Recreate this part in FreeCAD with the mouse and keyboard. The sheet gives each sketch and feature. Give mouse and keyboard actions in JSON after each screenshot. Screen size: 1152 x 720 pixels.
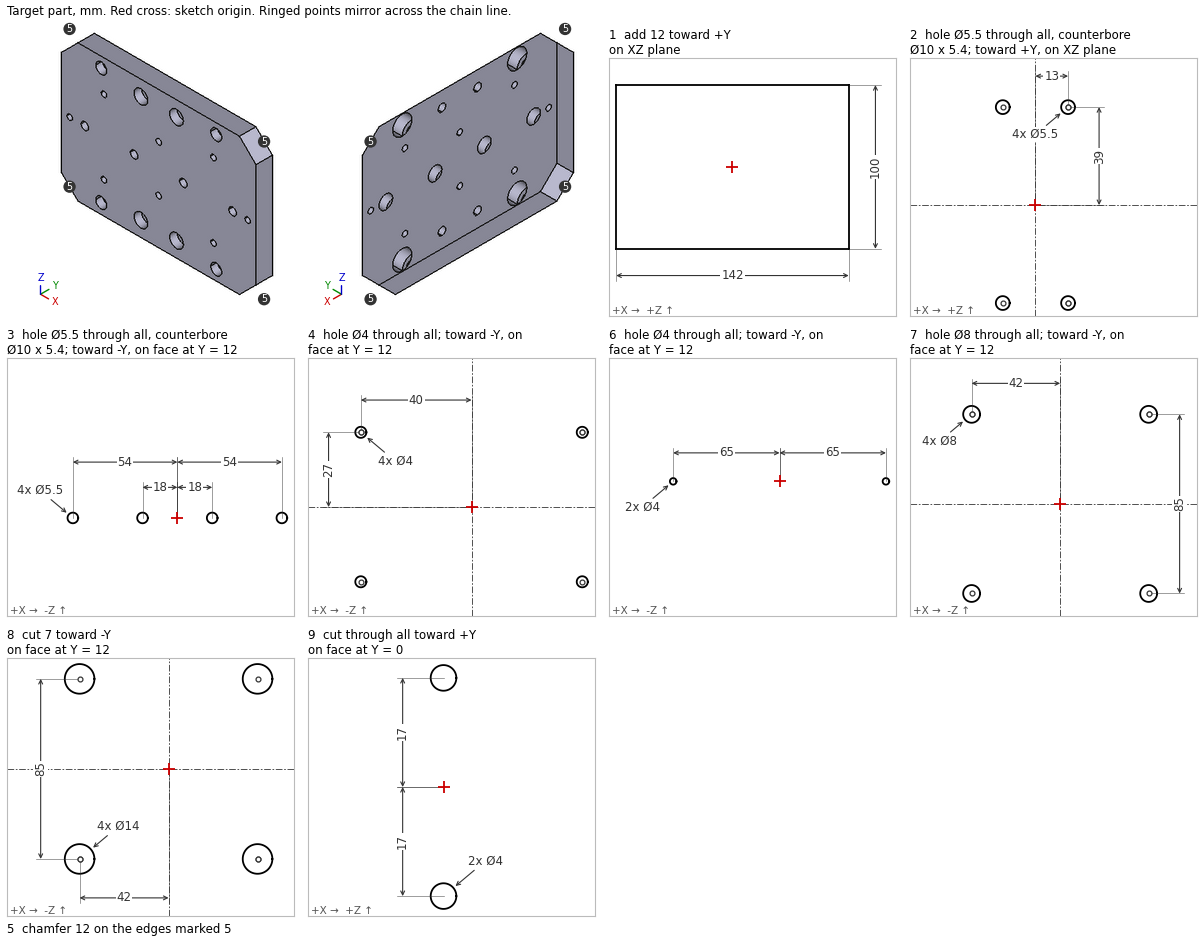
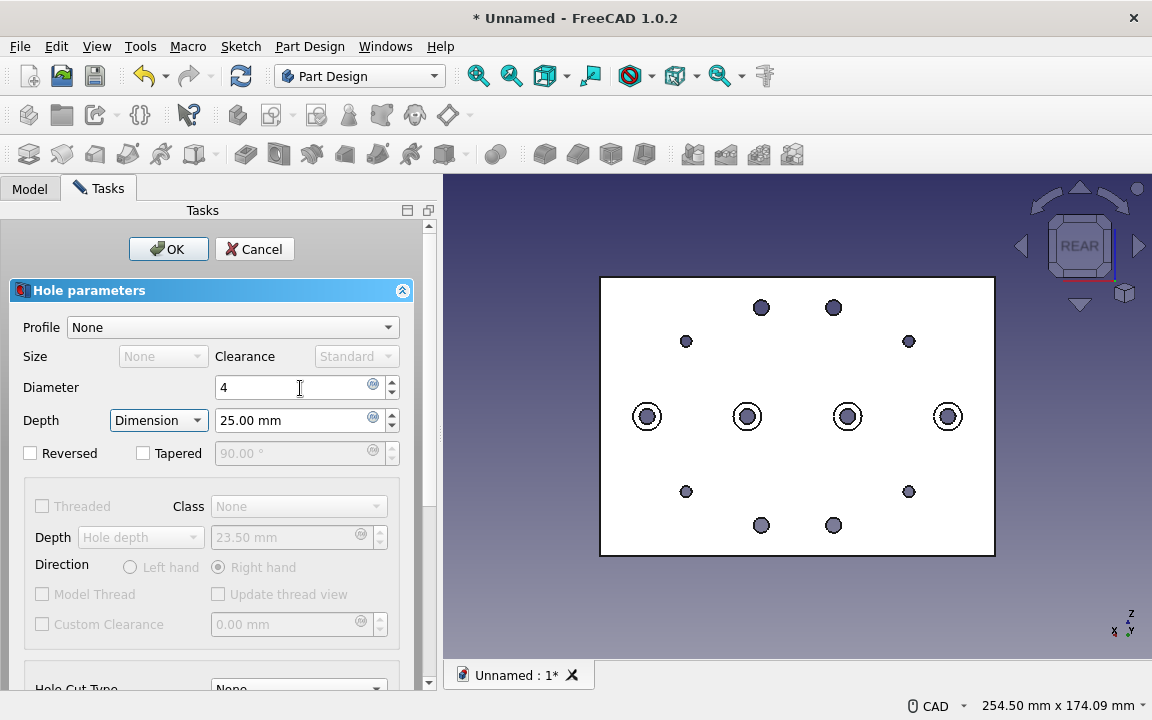
{"action": "left_click", "coordinate": [160, 420]}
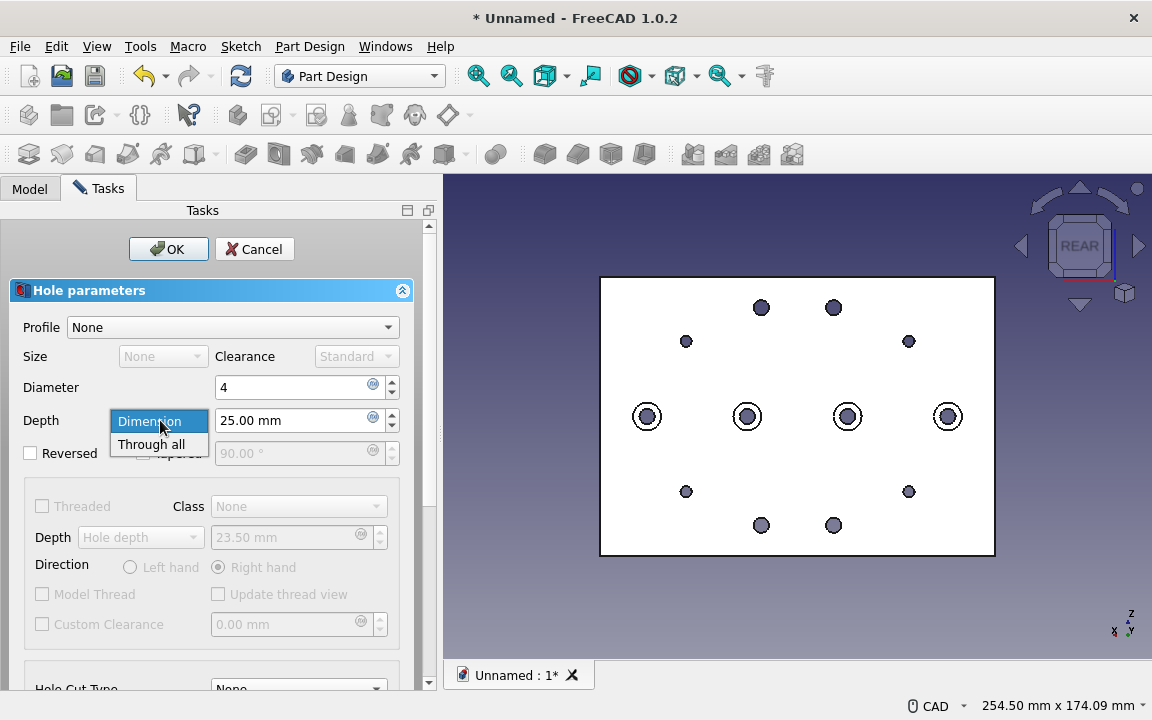
{"action": "left_click", "coordinate": [158, 444]}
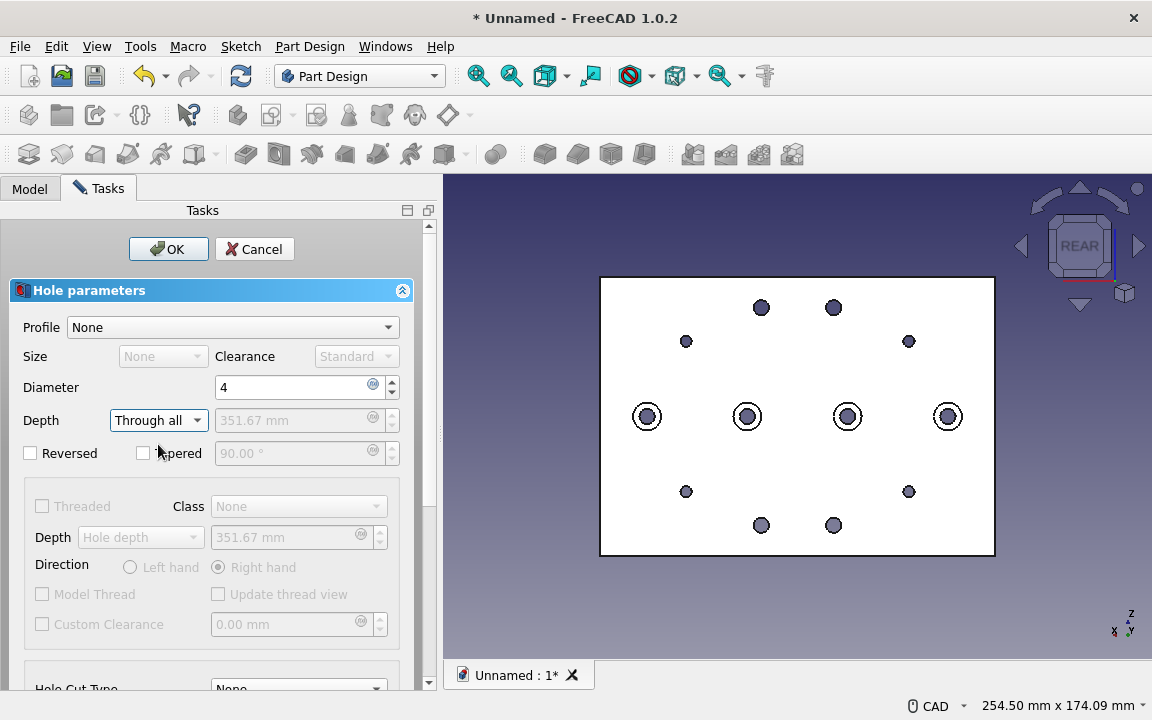
{"action": "left_click", "coordinate": [169, 249]}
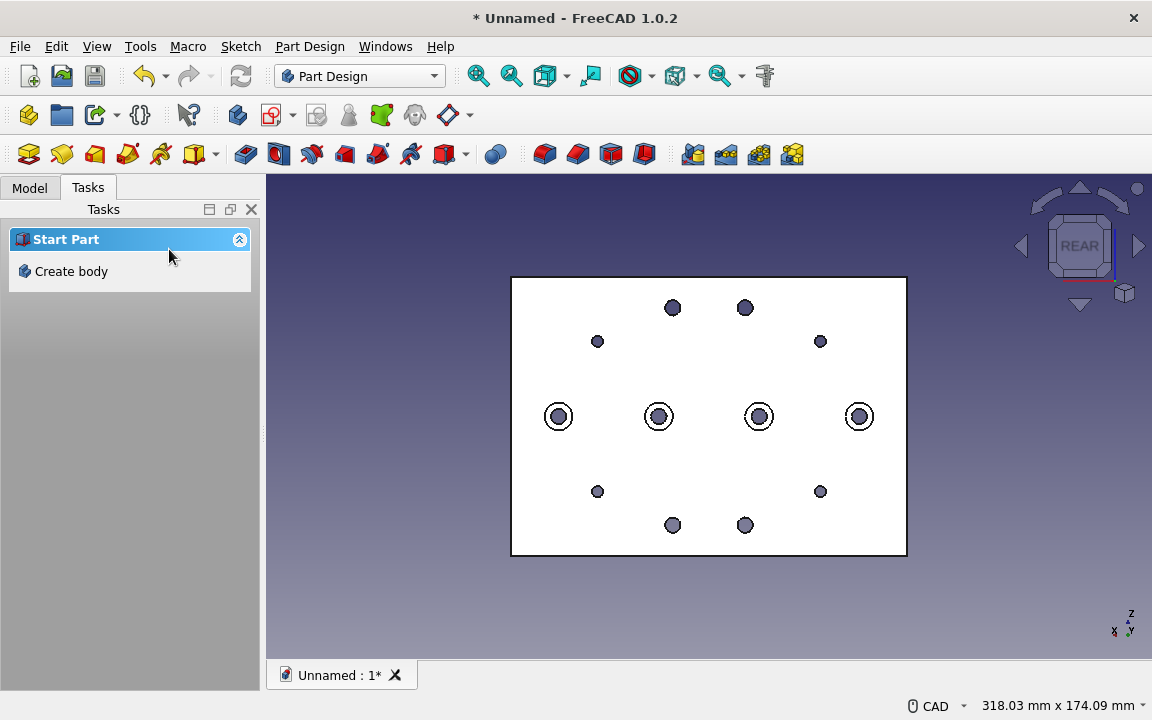
{"action": "key", "text": "0"}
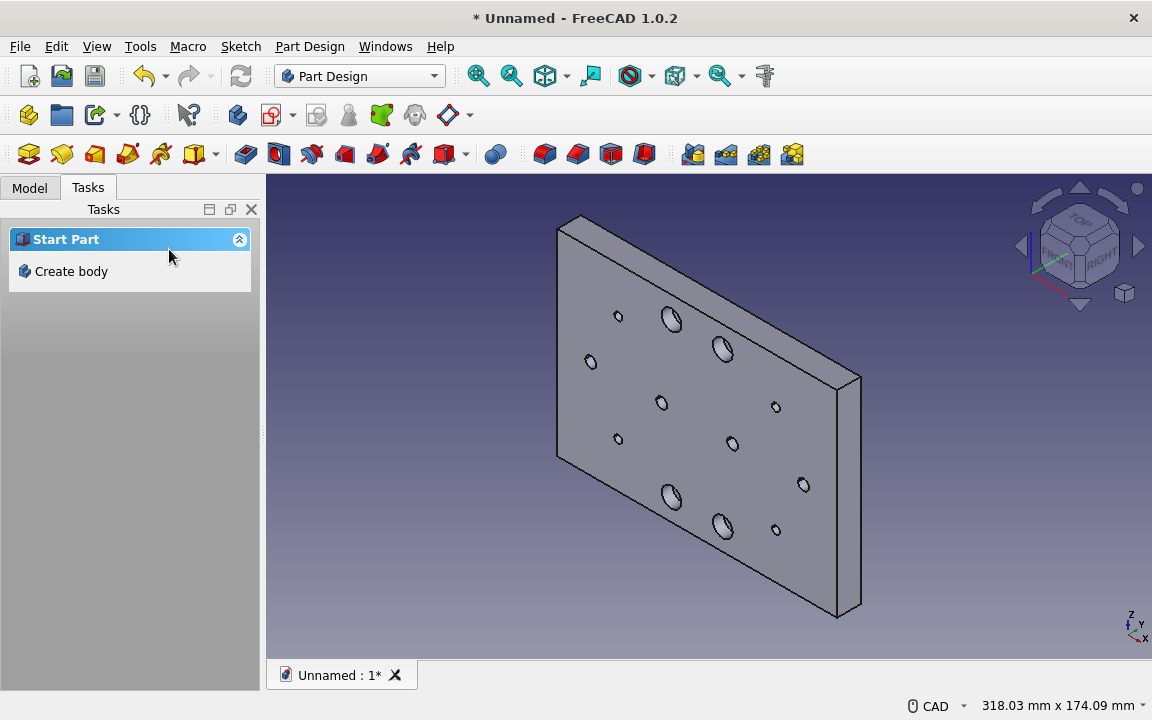
{"action": "left_click", "coordinate": [849, 383]}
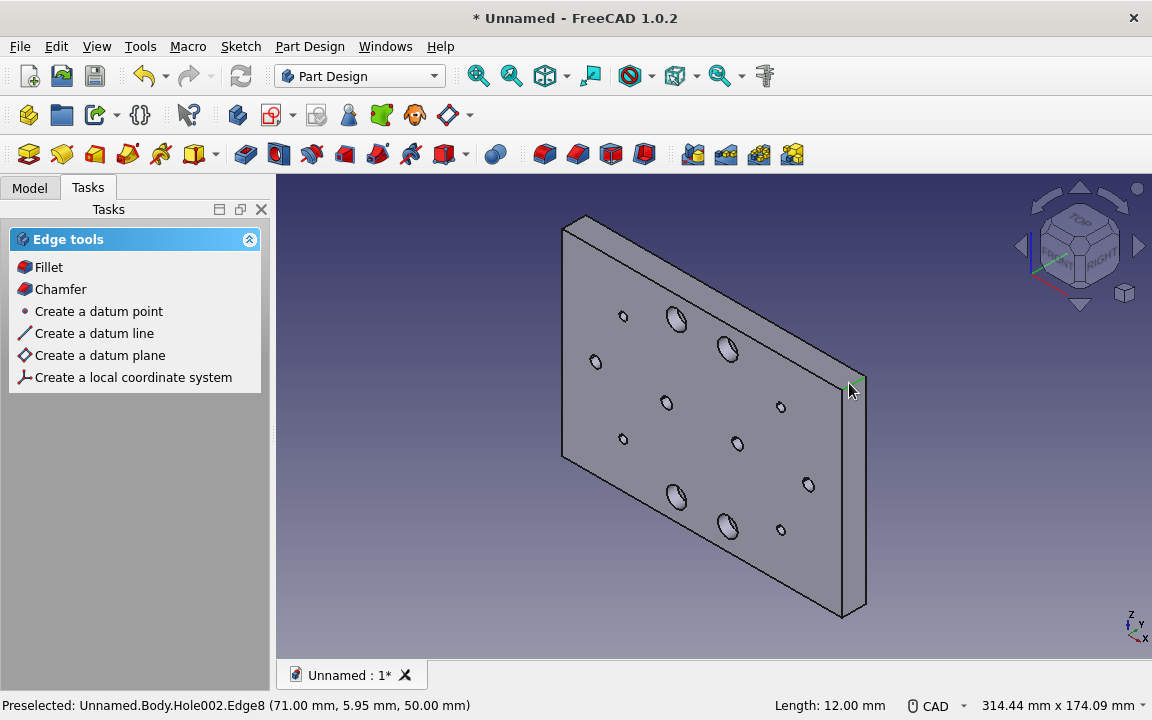
{"action": "key", "text": "2"}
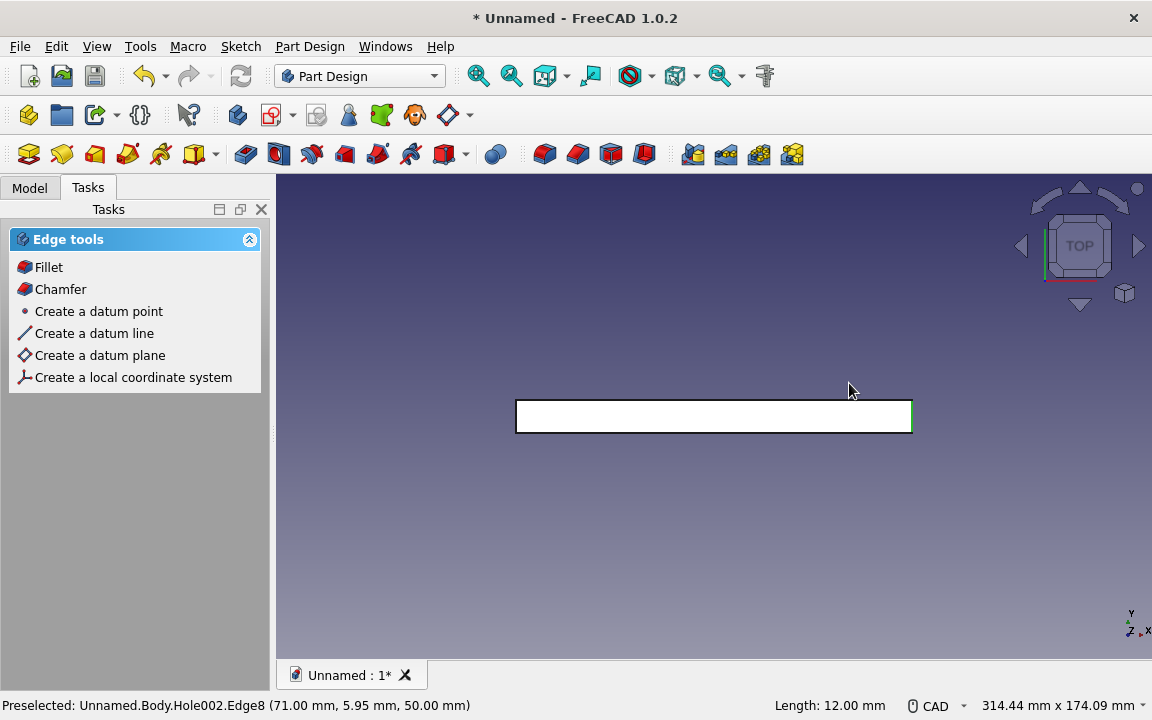
{"action": "left_click", "coordinate": [516, 415], "text": "ctrl"}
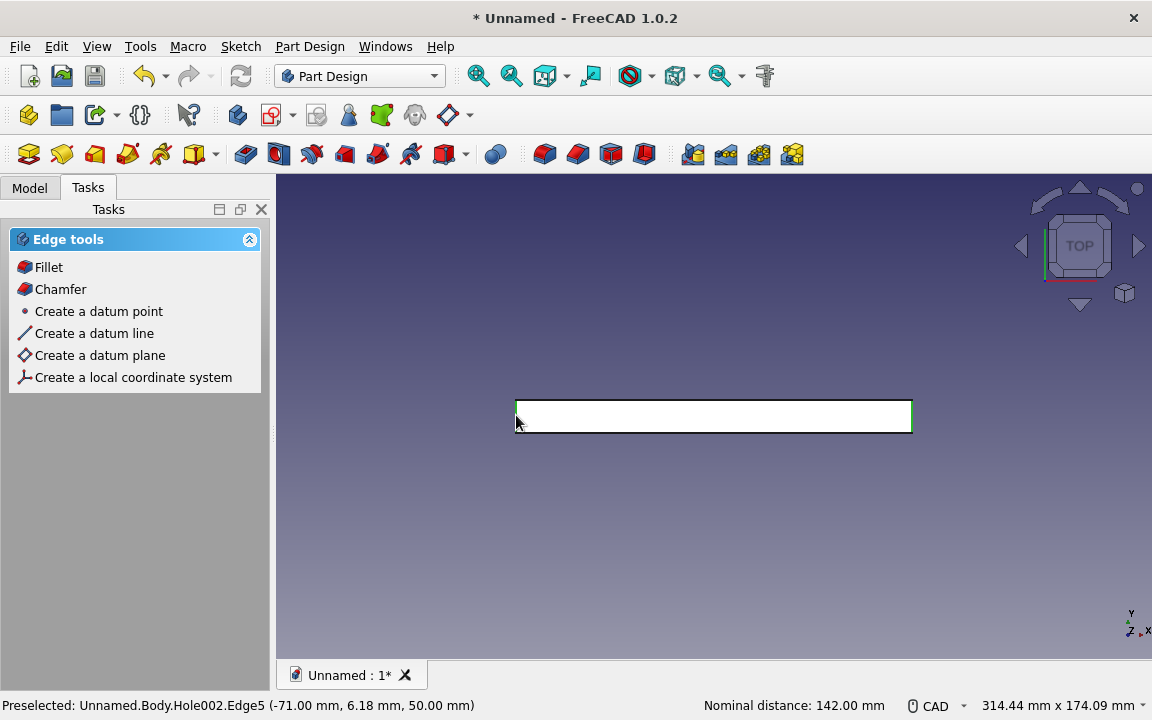
{"action": "key", "text": "1"}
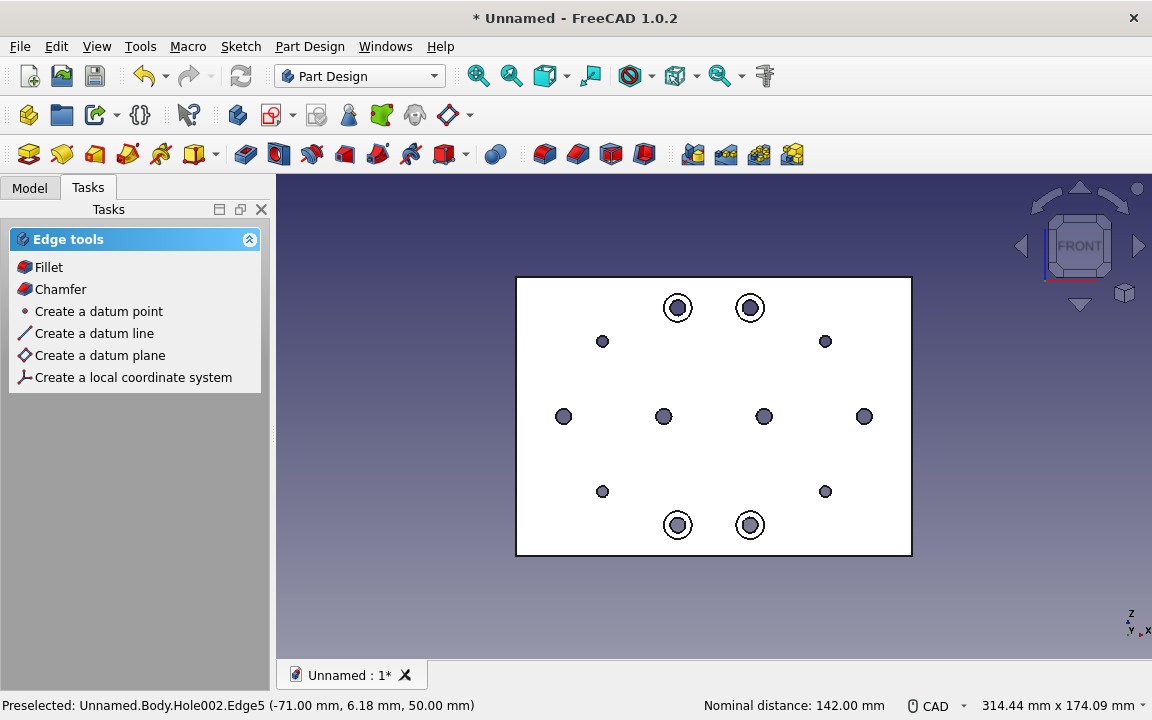
{"action": "key", "text": "3"}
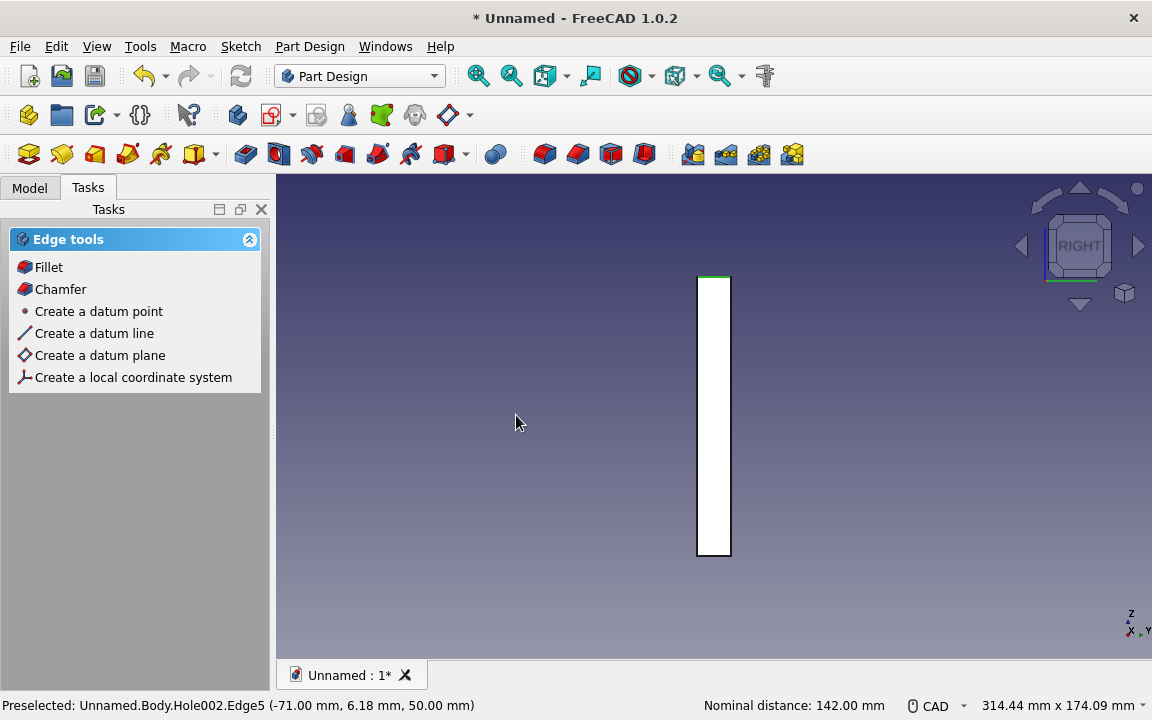
{"action": "left_click", "coordinate": [714, 555], "text": "ctrl"}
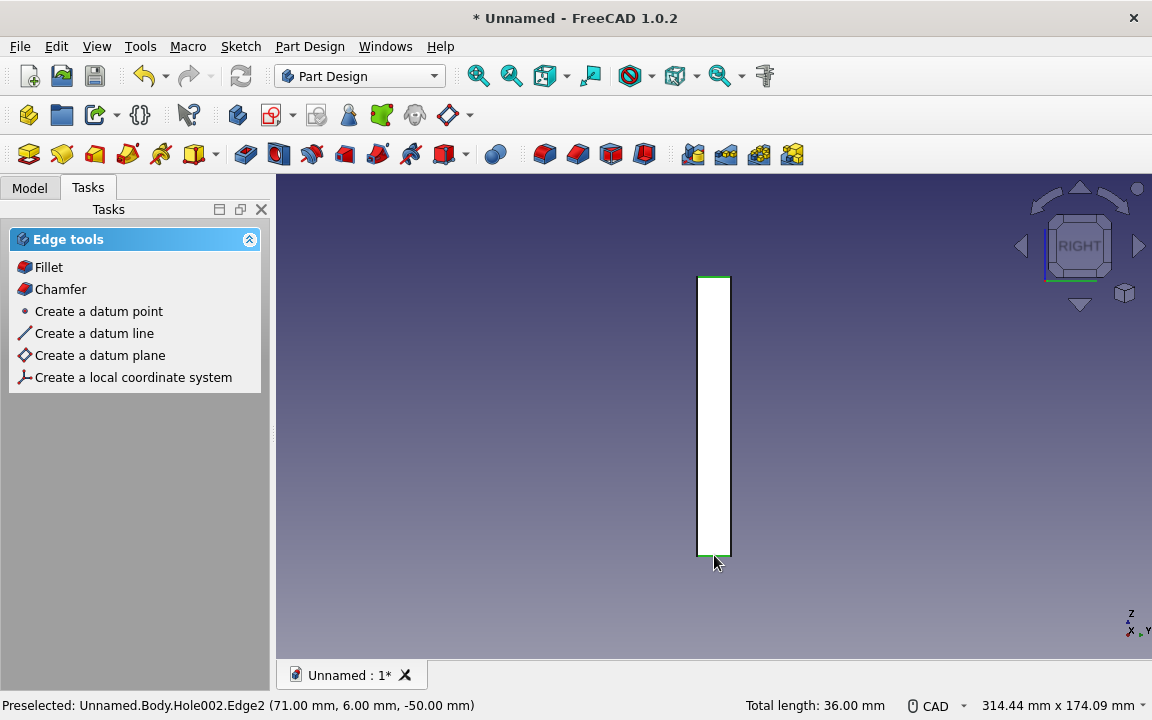
{"action": "key", "text": "5"}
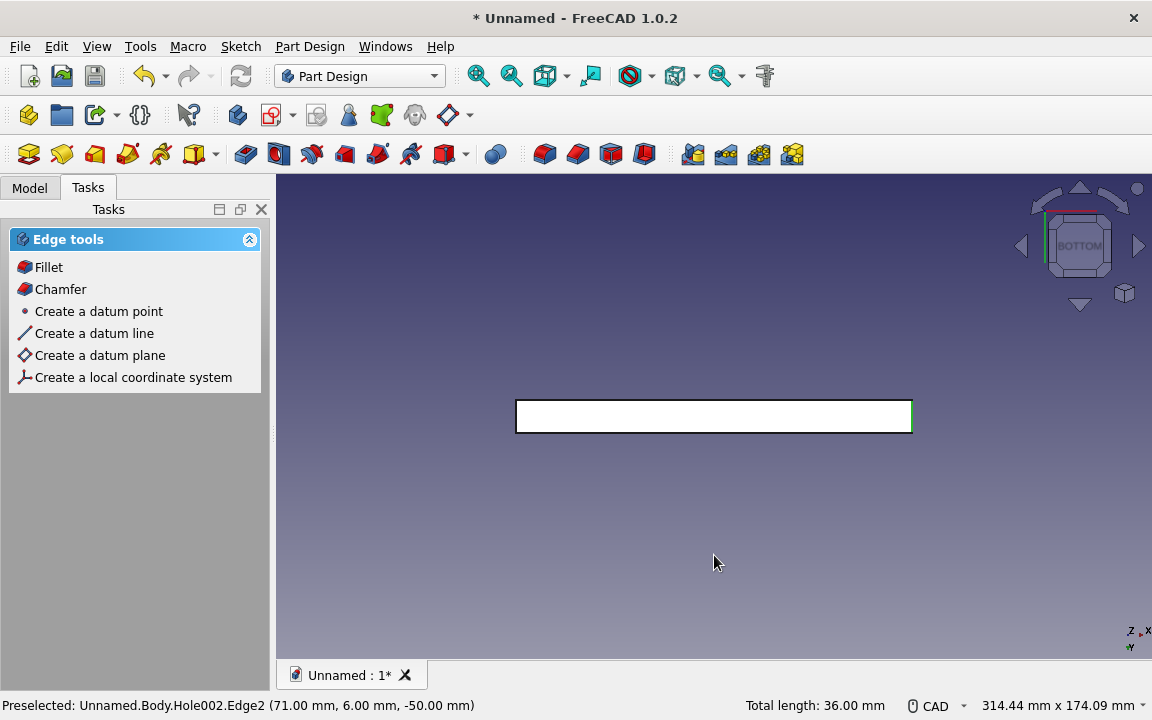
{"action": "left_click", "coordinate": [516, 416], "text": "ctrl"}